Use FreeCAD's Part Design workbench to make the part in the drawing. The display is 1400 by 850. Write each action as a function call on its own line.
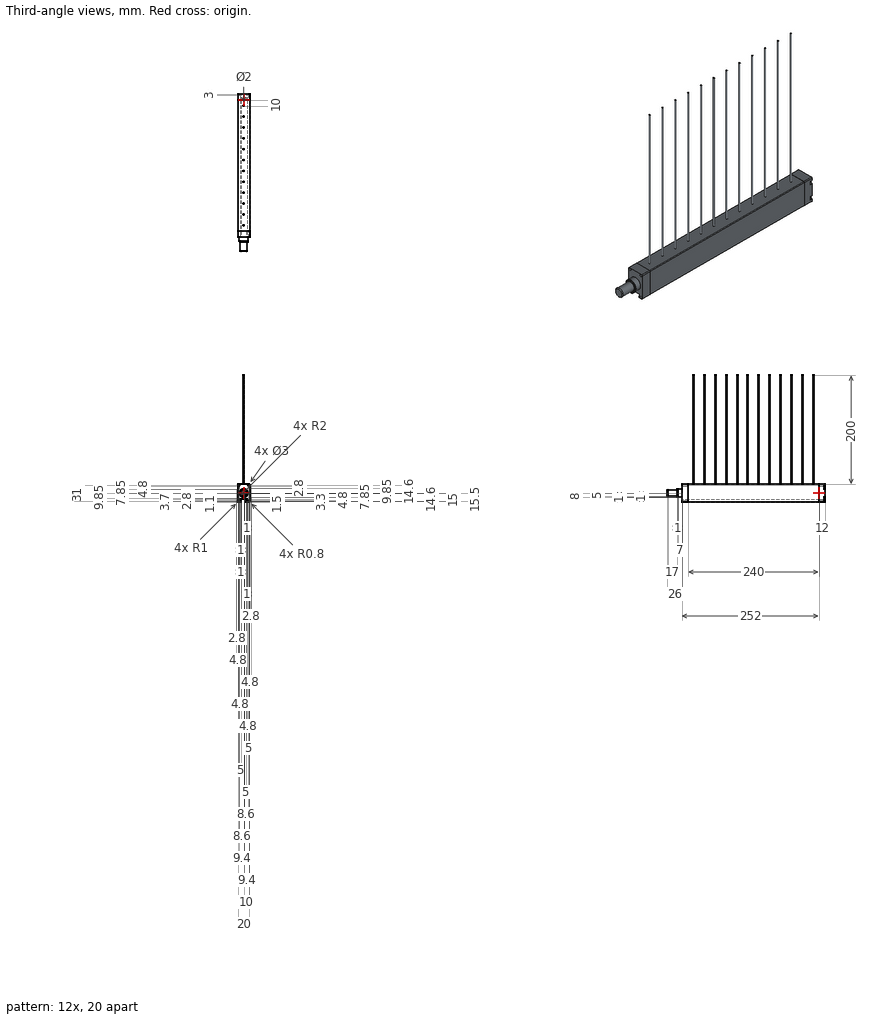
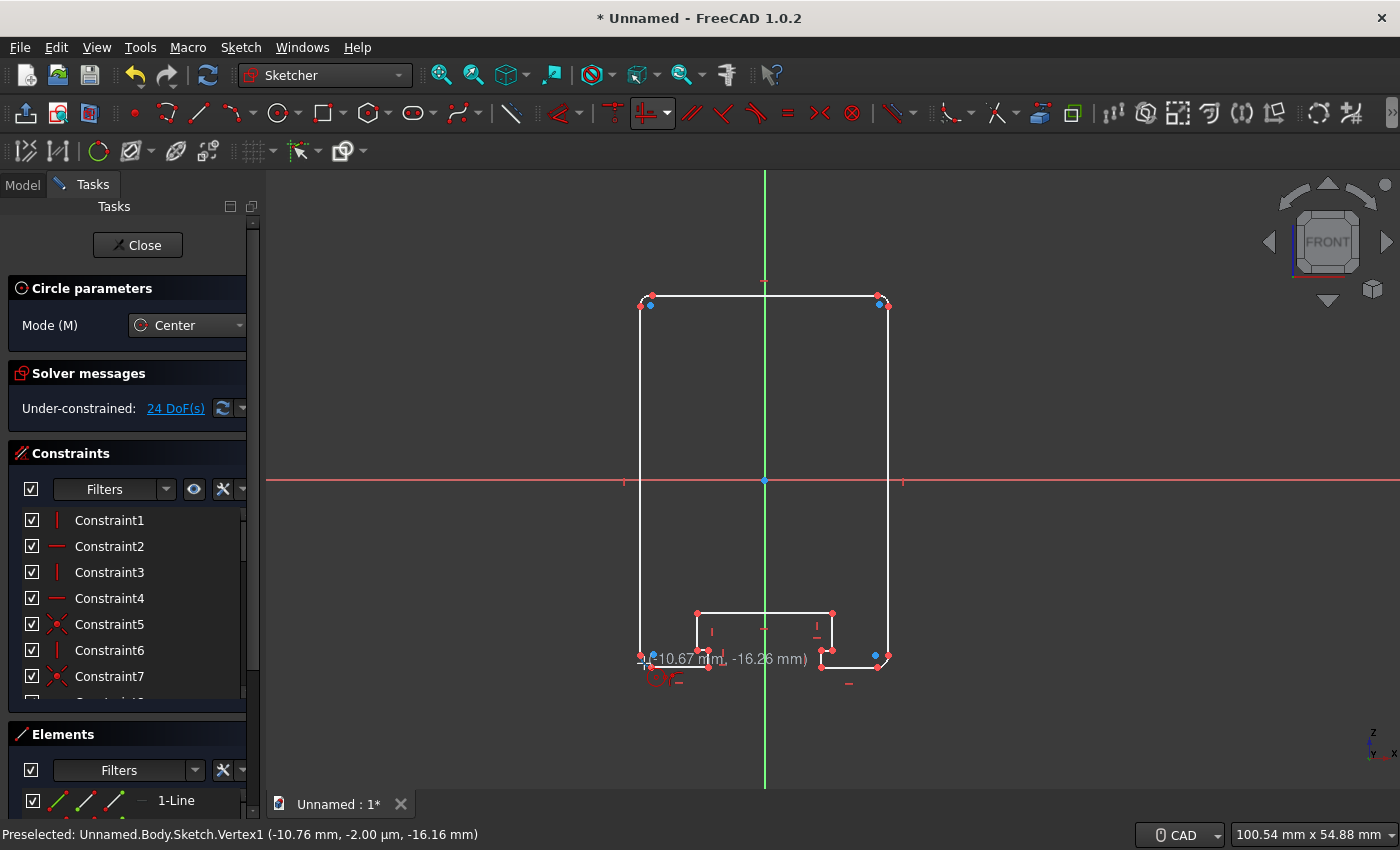
scroll(862, 316, up, 2)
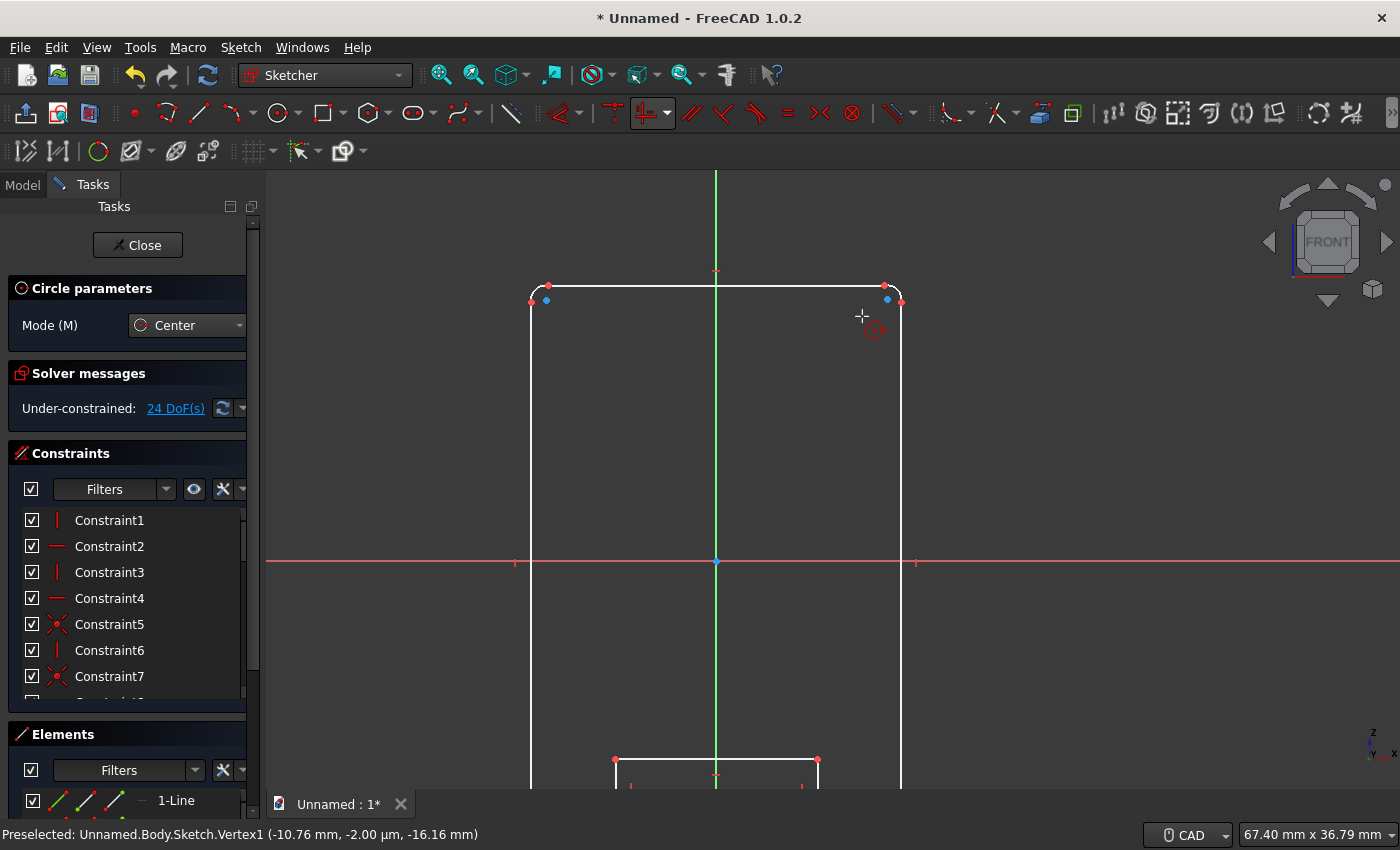
click(861, 316)
click(843, 298)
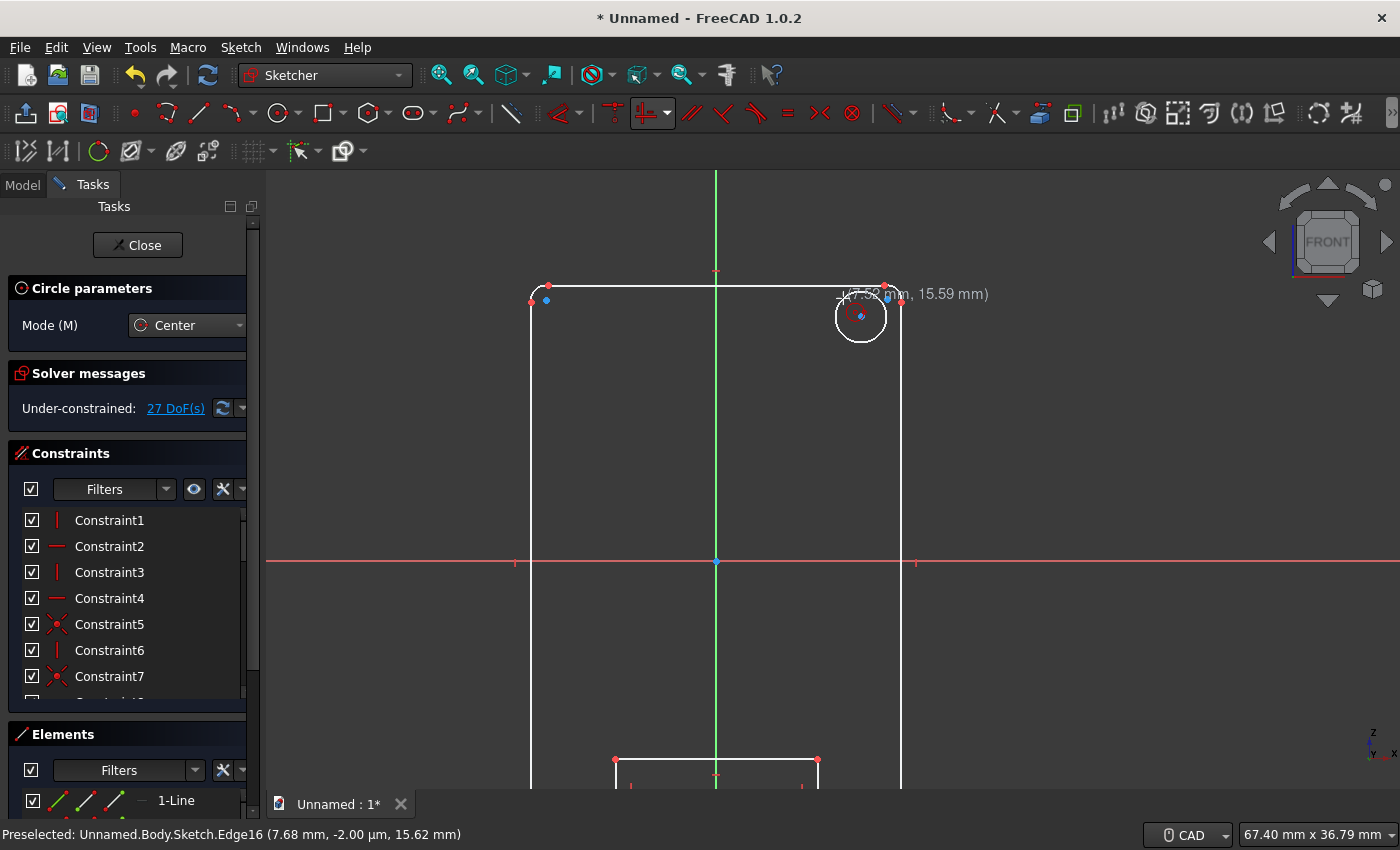
click(572, 316)
click(590, 298)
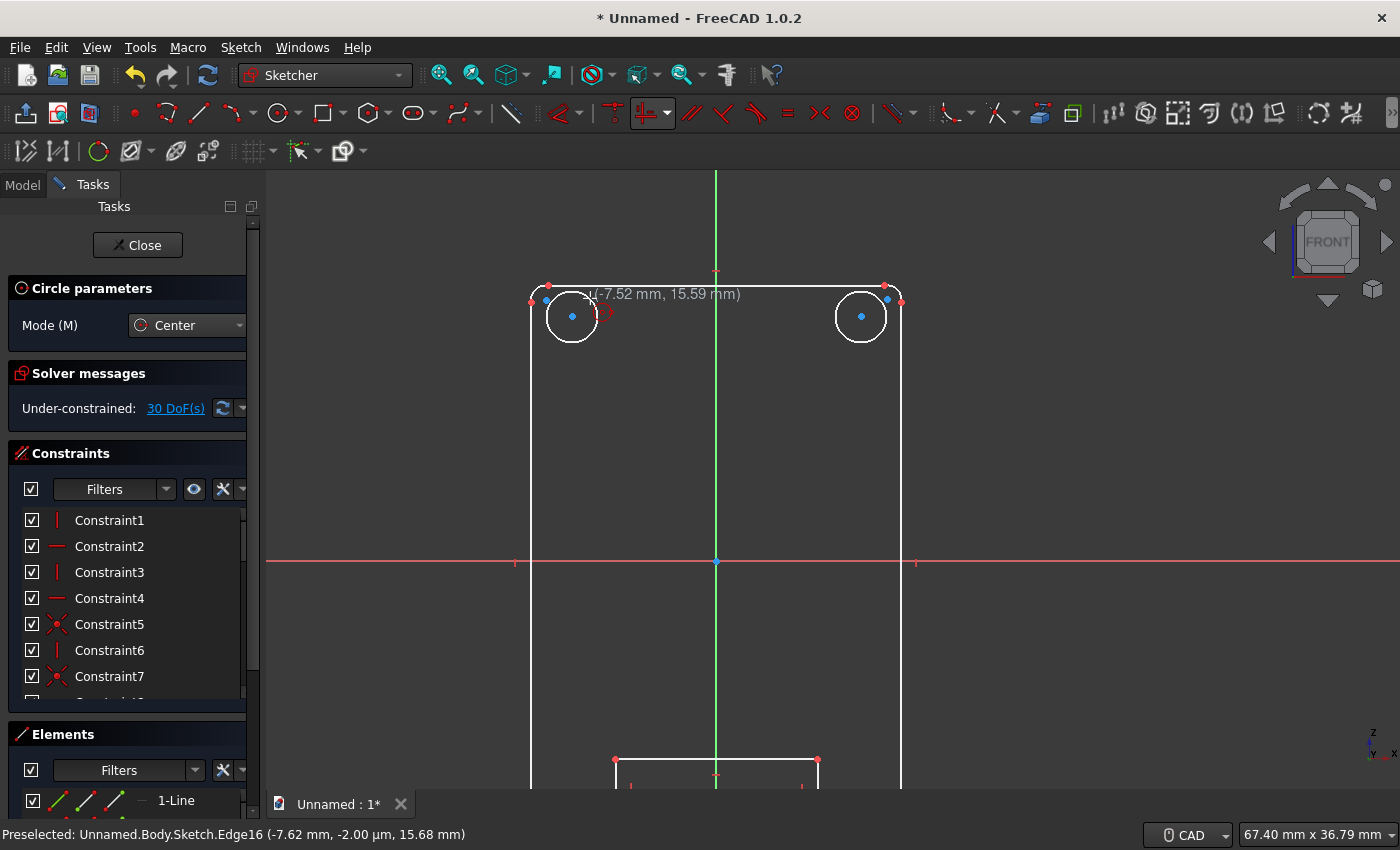
scroll(862, 313, down, 2)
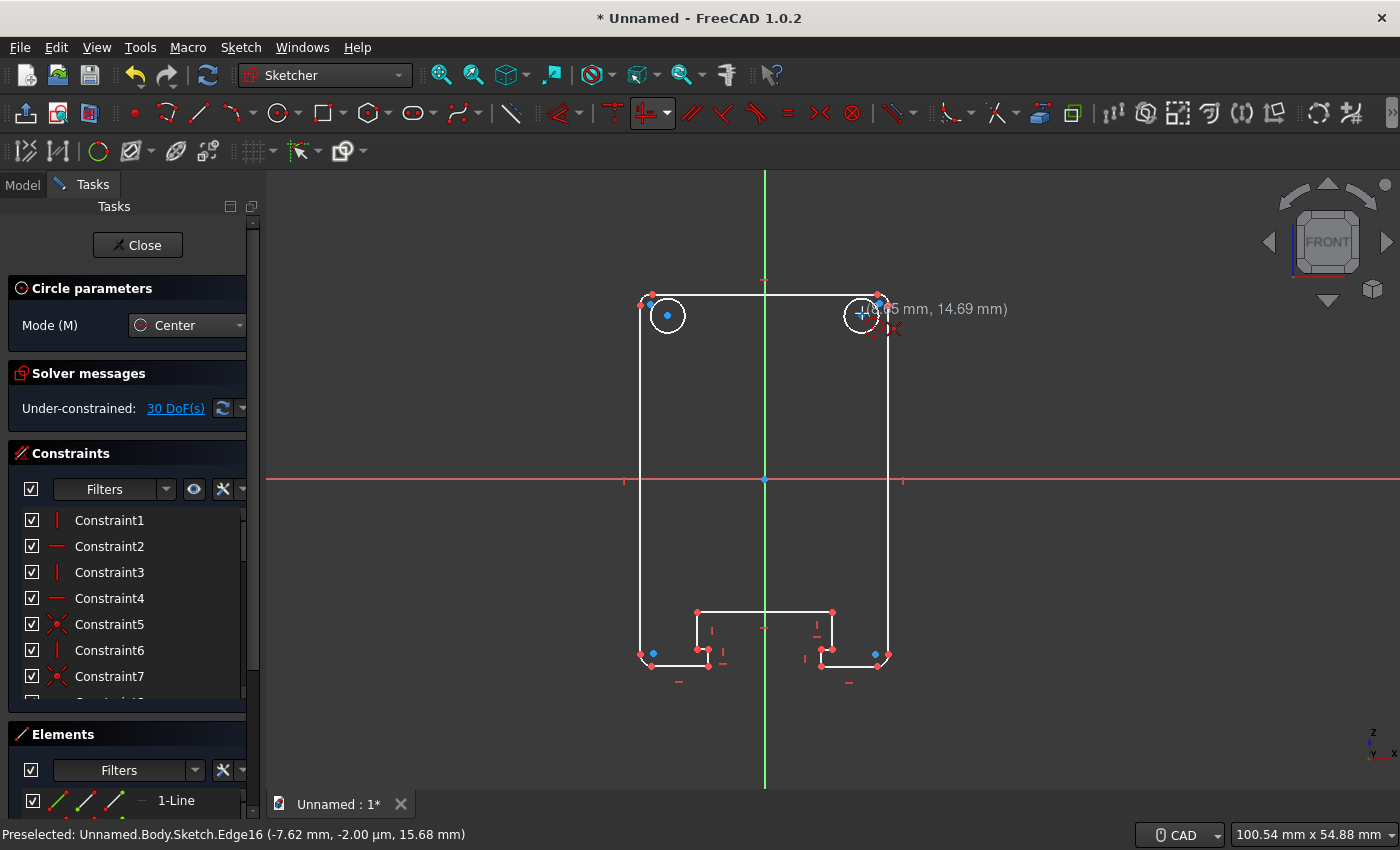
scroll(862, 644, up, 2)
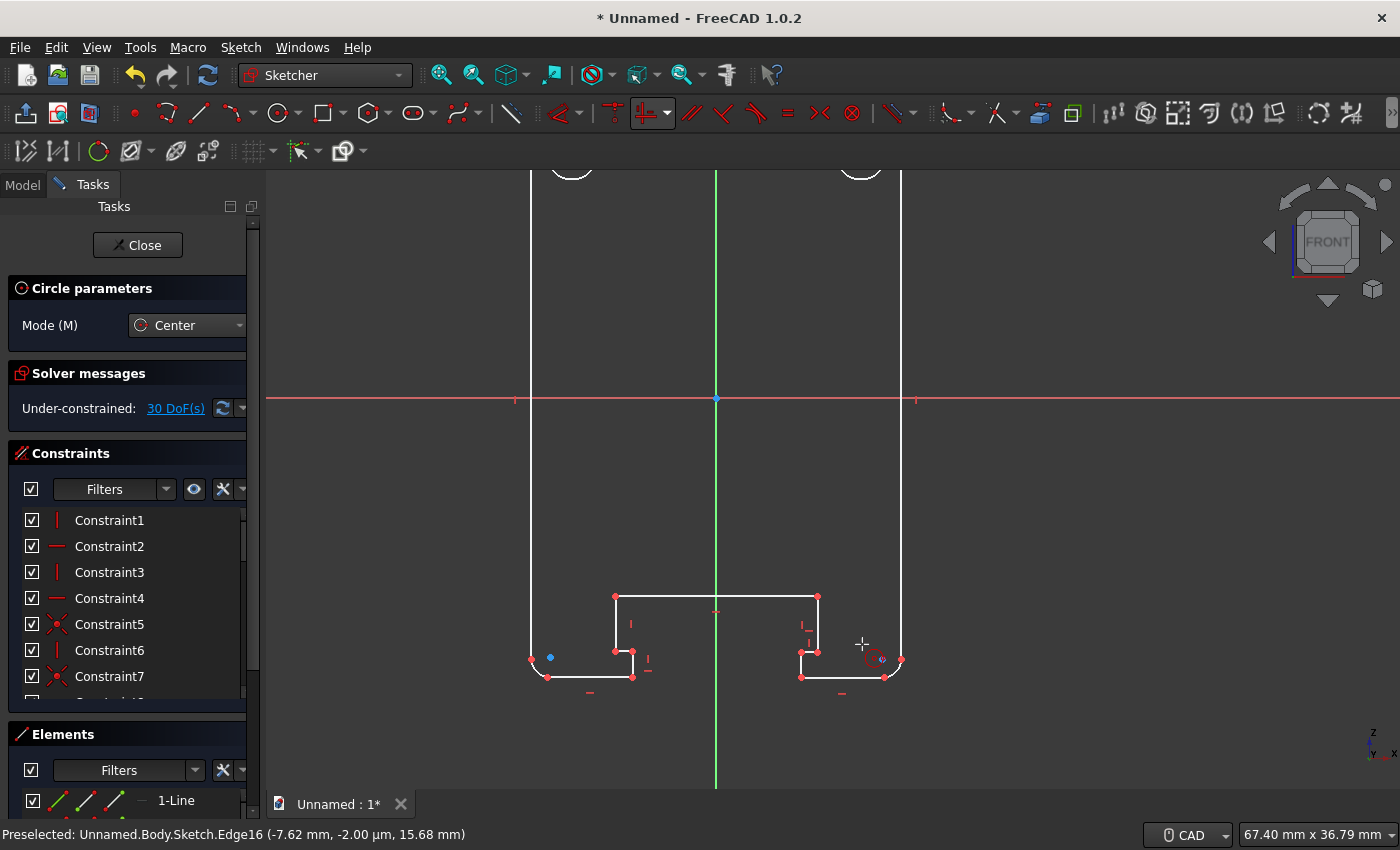
click(861, 644)
click(879, 626)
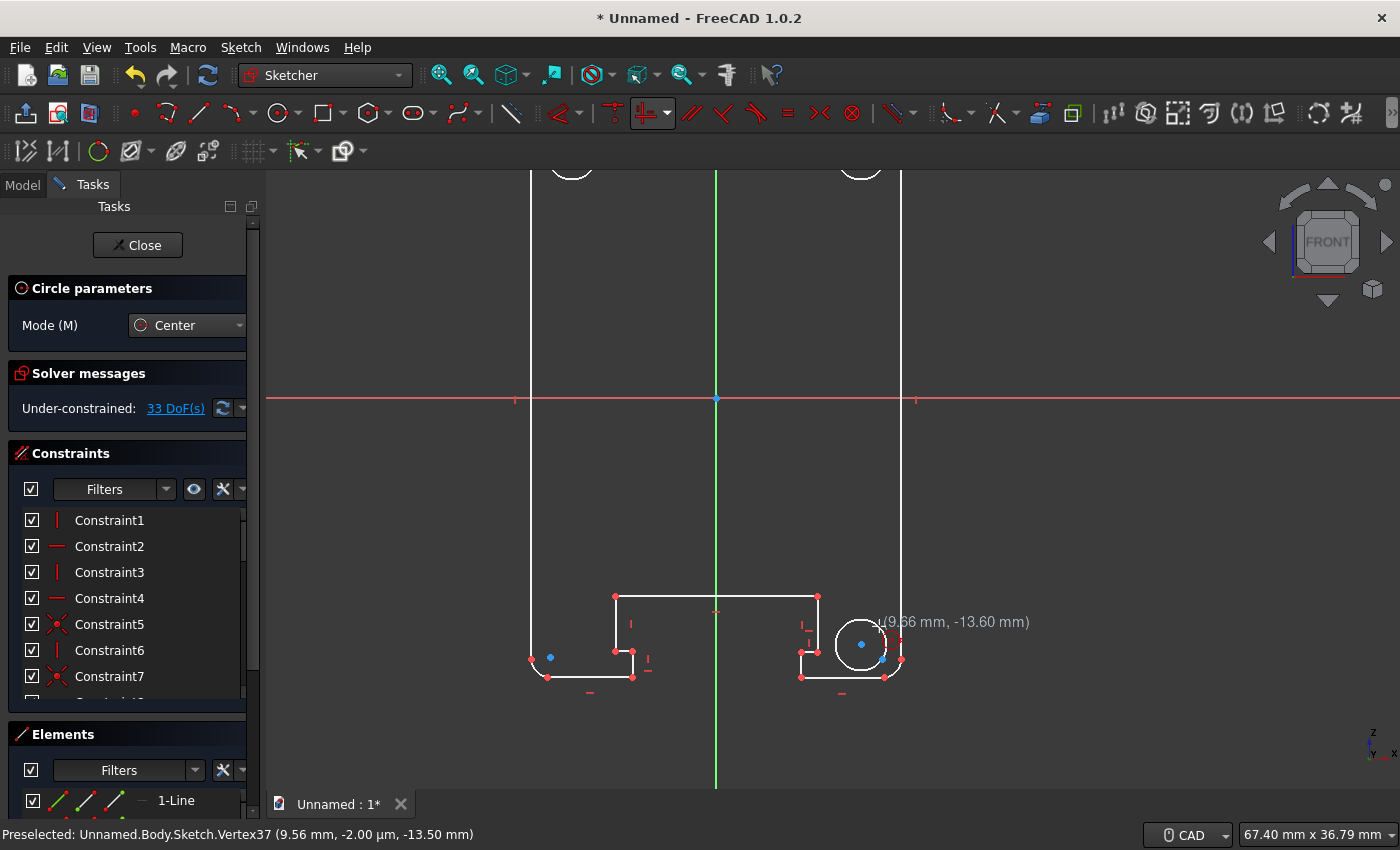
click(572, 644)
click(590, 626)
key(Escape)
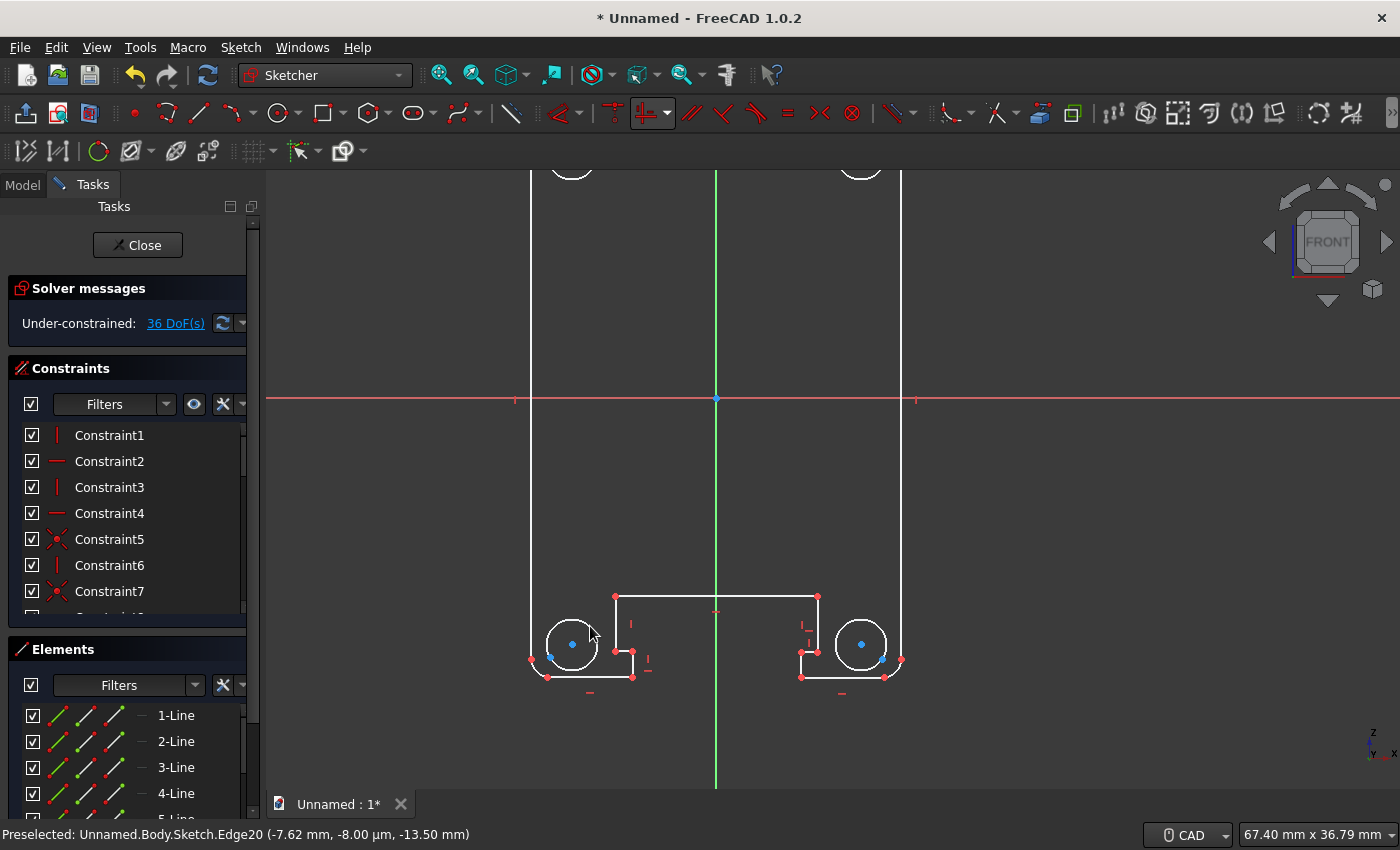
click(531, 504)